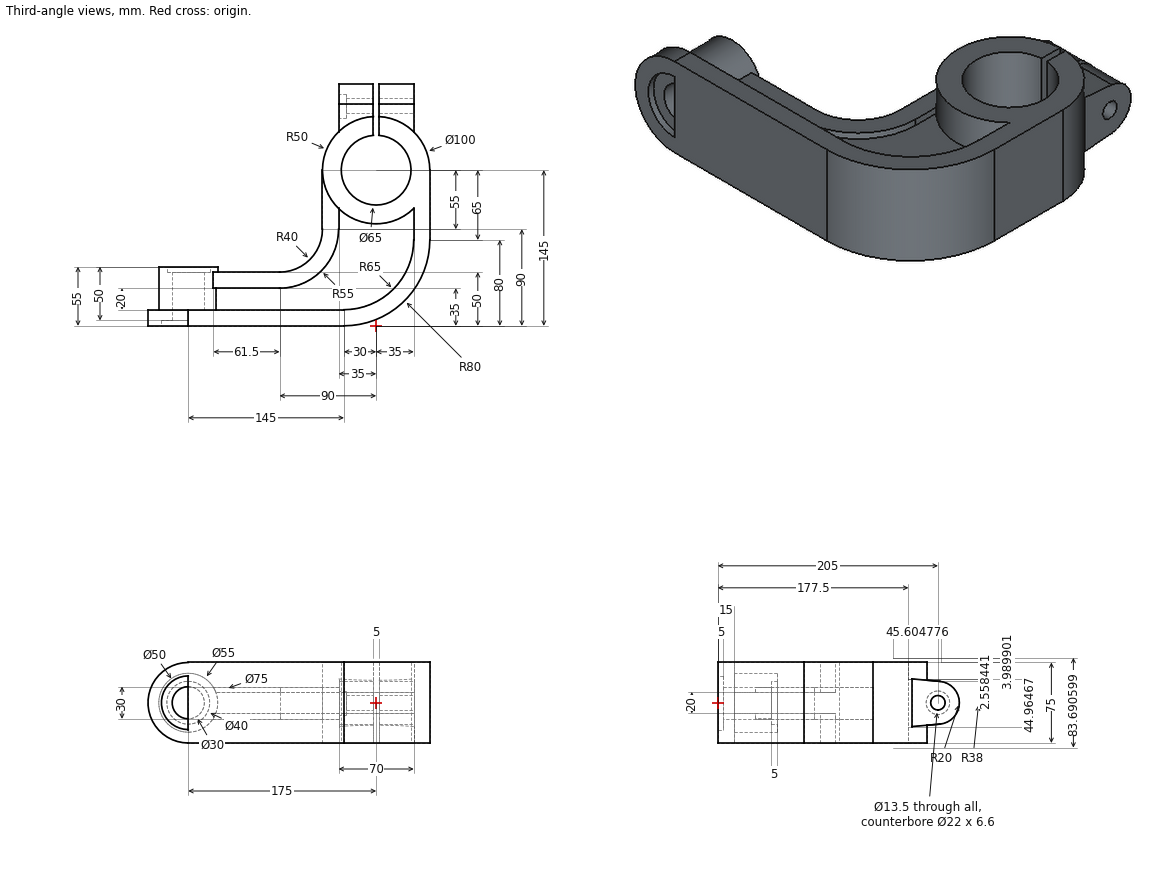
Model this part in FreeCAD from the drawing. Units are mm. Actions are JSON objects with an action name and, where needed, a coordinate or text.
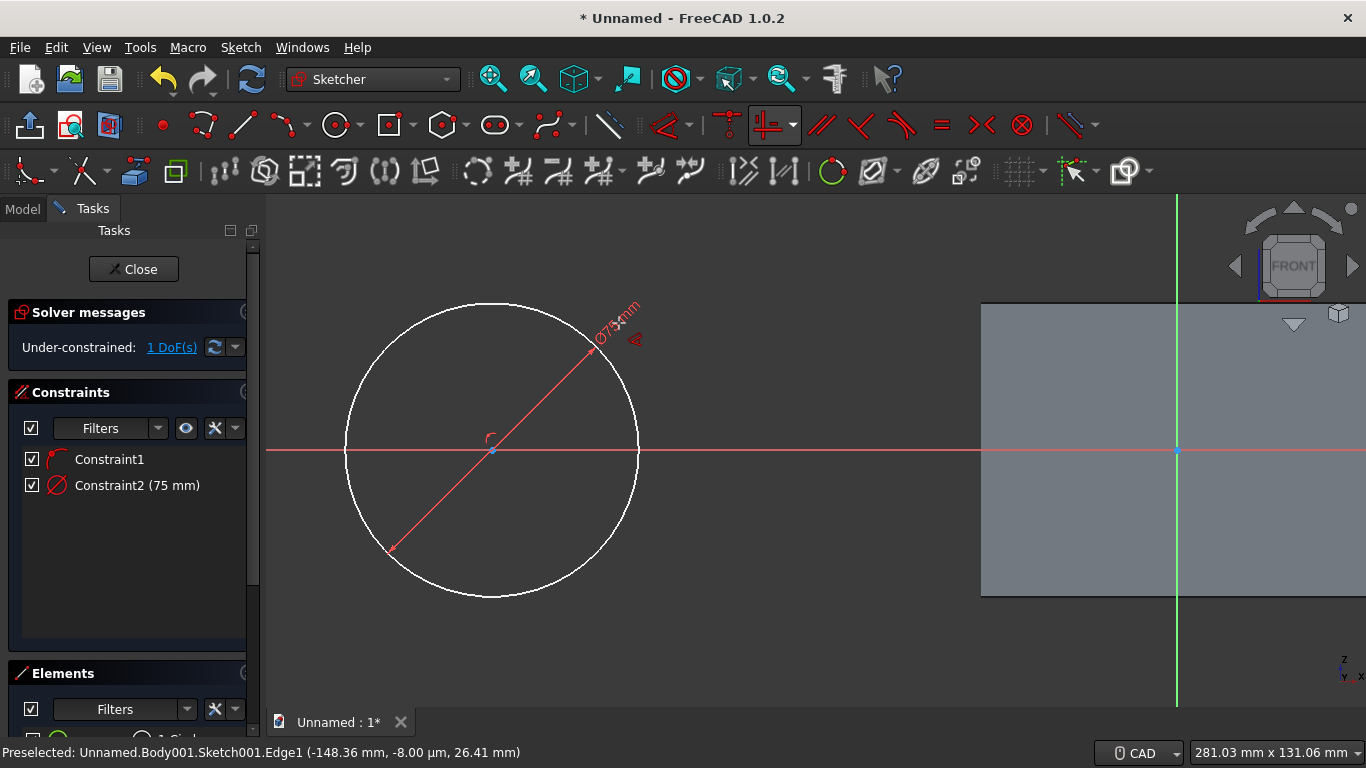
{"action": "left_click", "coordinate": [492, 450]}
{"action": "left_click", "coordinate": [835, 484]}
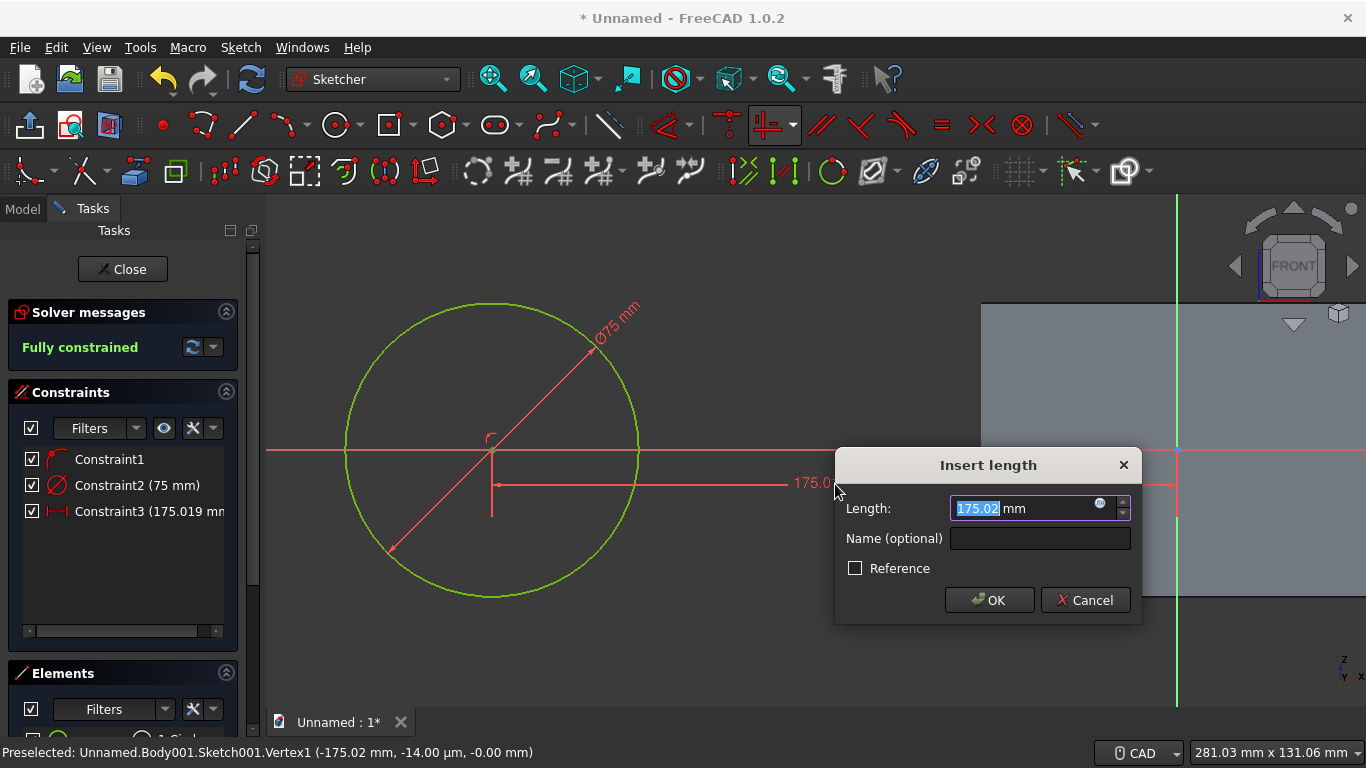
{"action": "type", "text": "175"}
{"action": "key", "text": "Return"}
{"action": "key", "text": "Escape"}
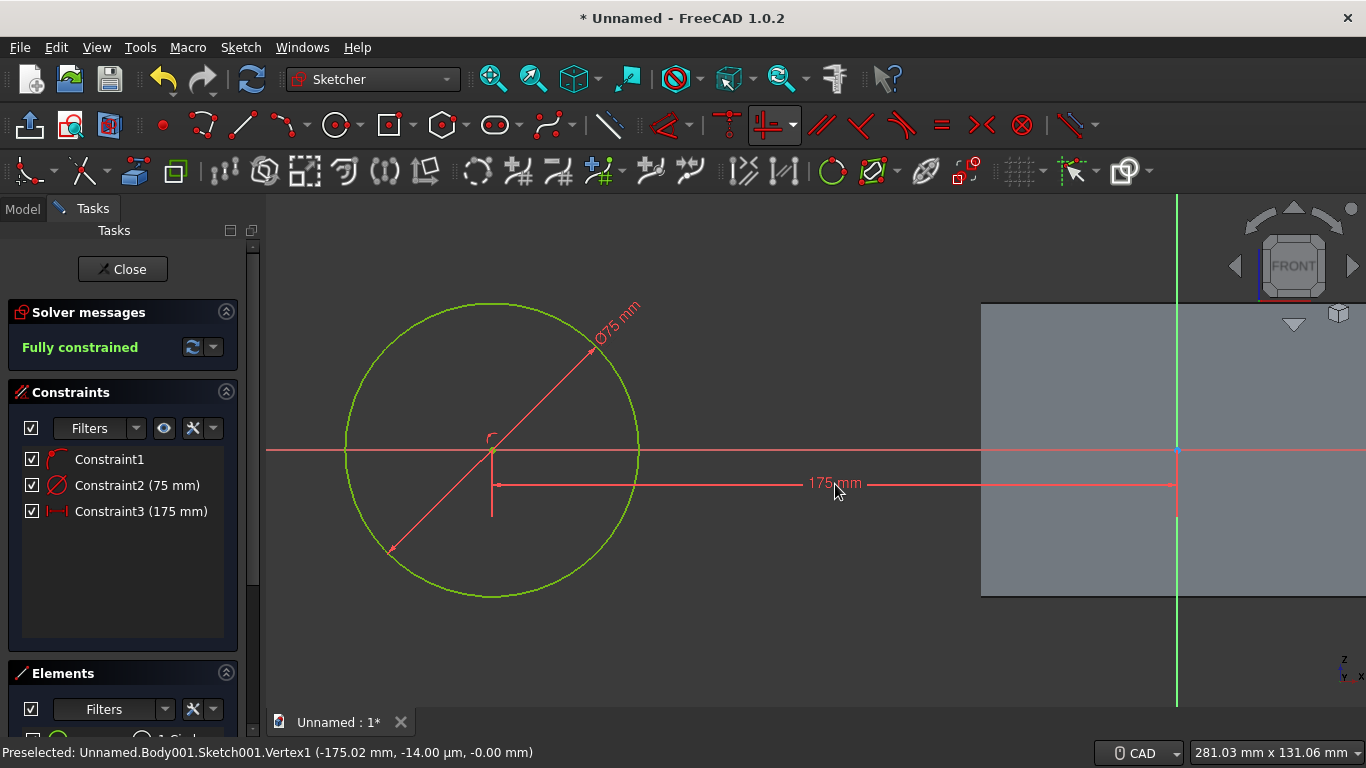
{"action": "left_click", "coordinate": [123, 269]}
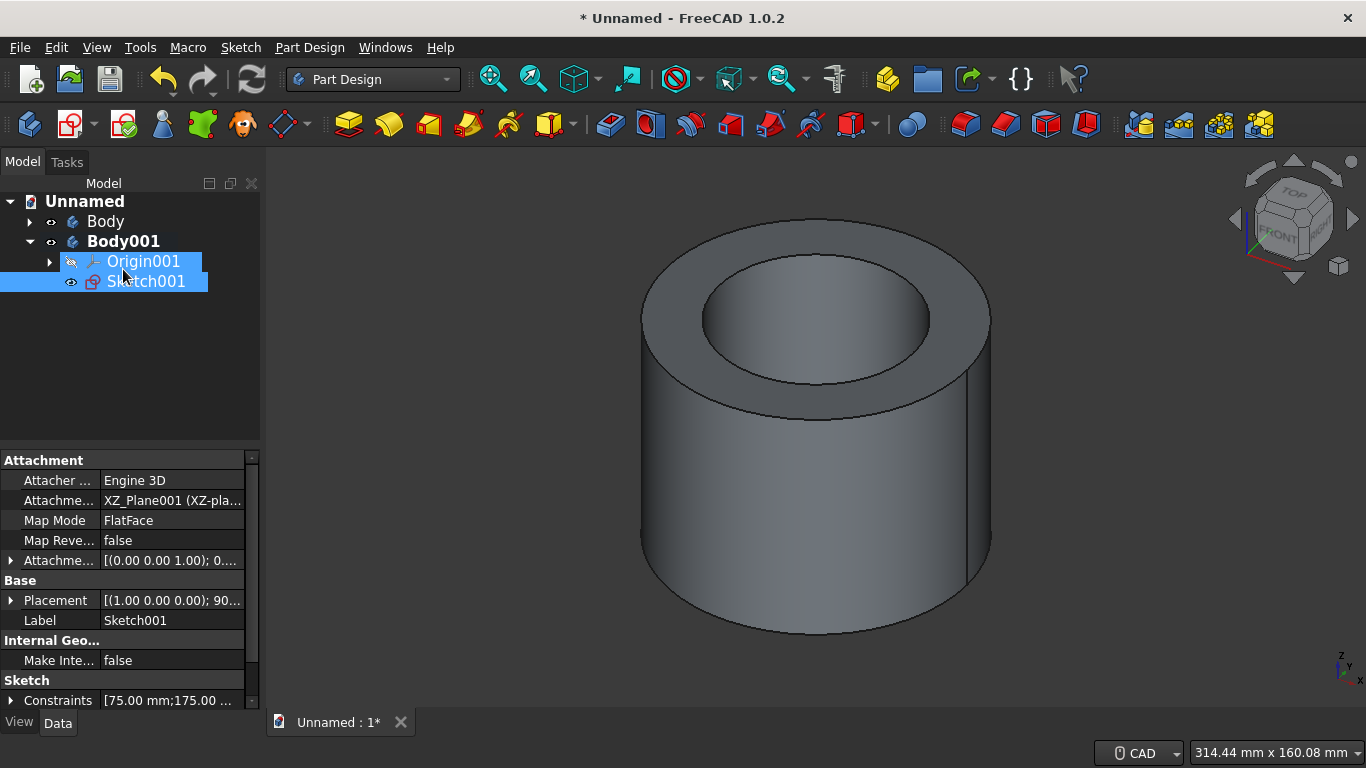
{"action": "left_click", "coordinate": [350, 124]}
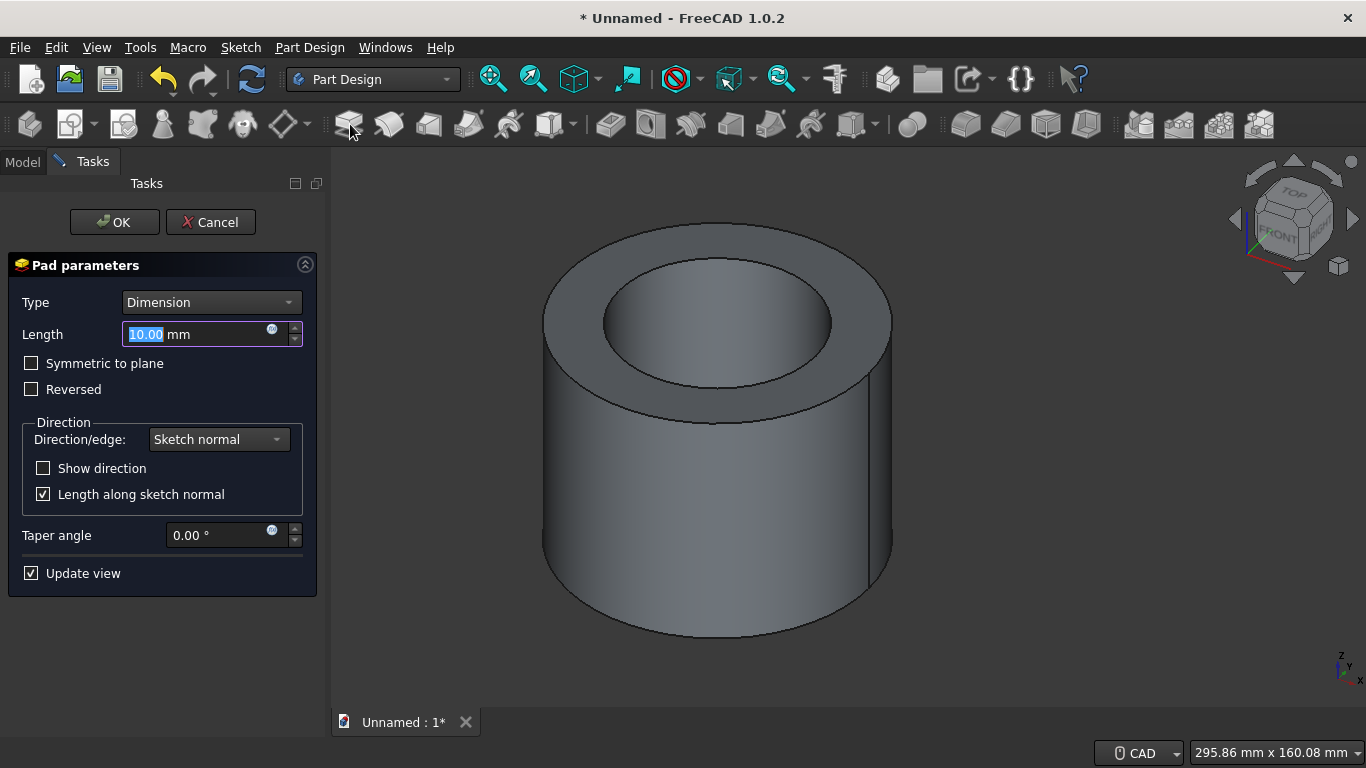
{"action": "type", "text": "15"}
{"action": "key", "text": "Tab"}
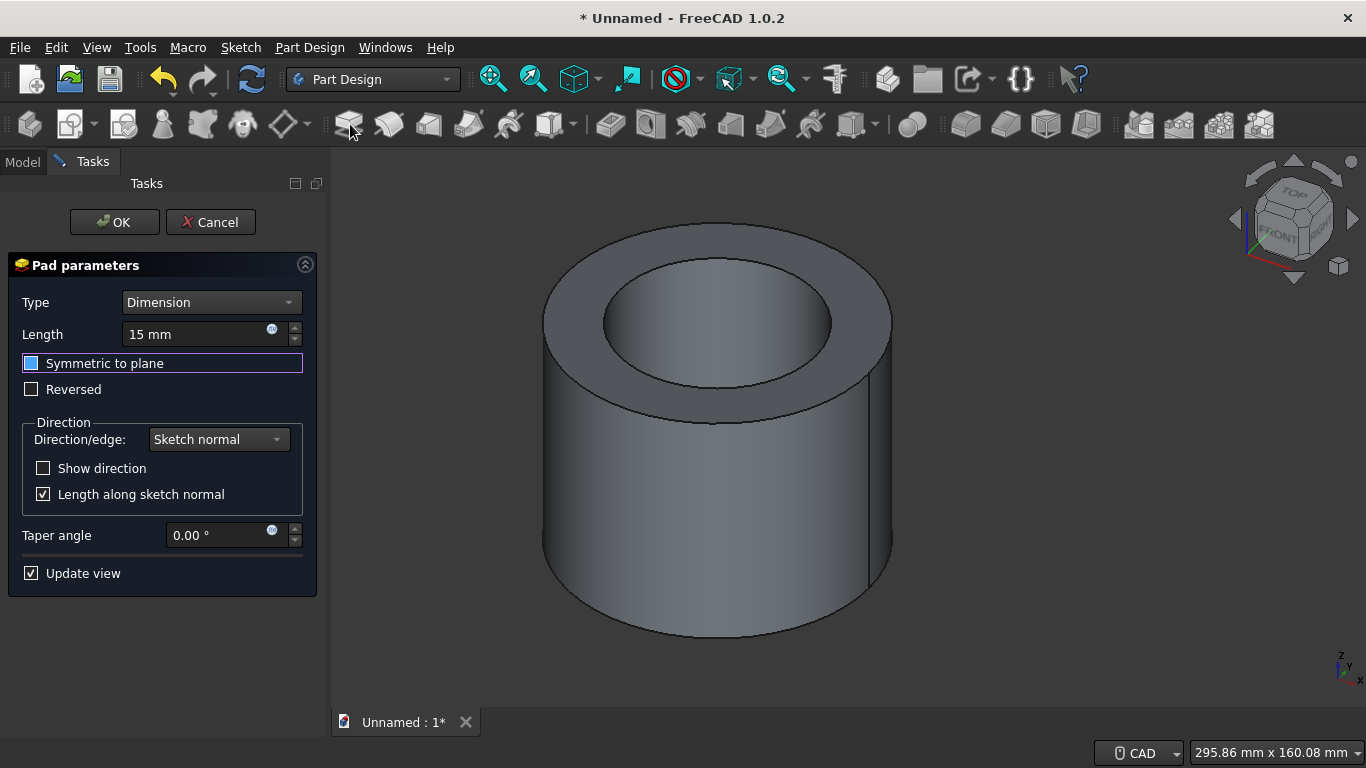
{"action": "left_click", "coordinate": [30, 389]}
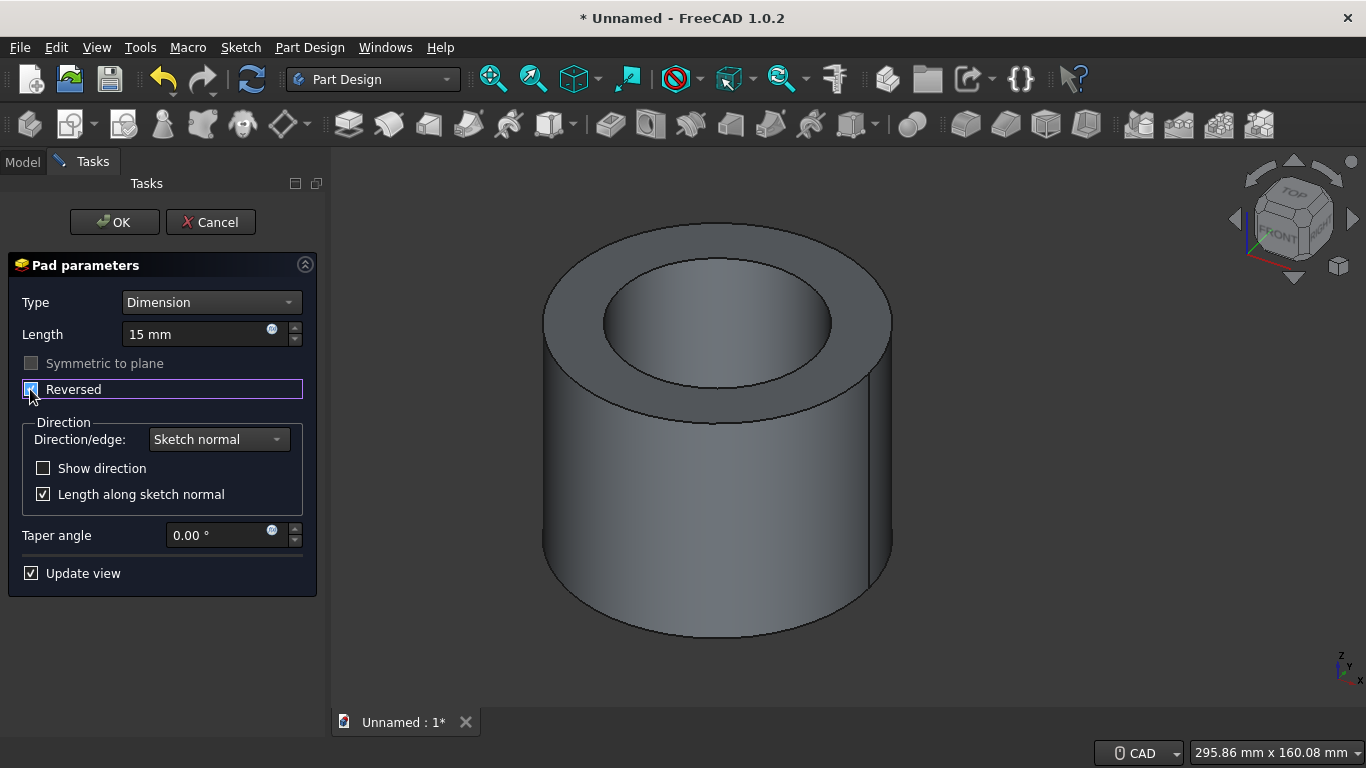
{"action": "left_click", "coordinate": [115, 222]}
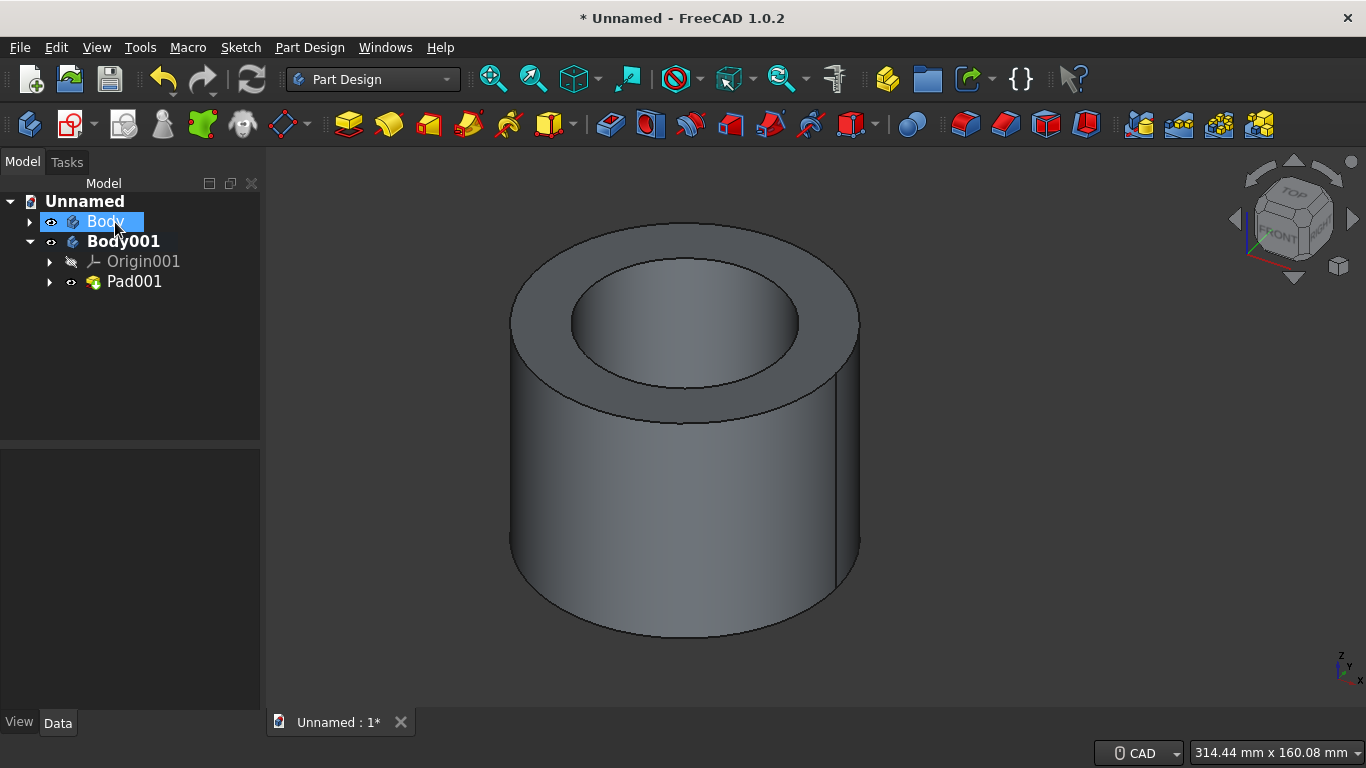
{"action": "key", "text": "v f"}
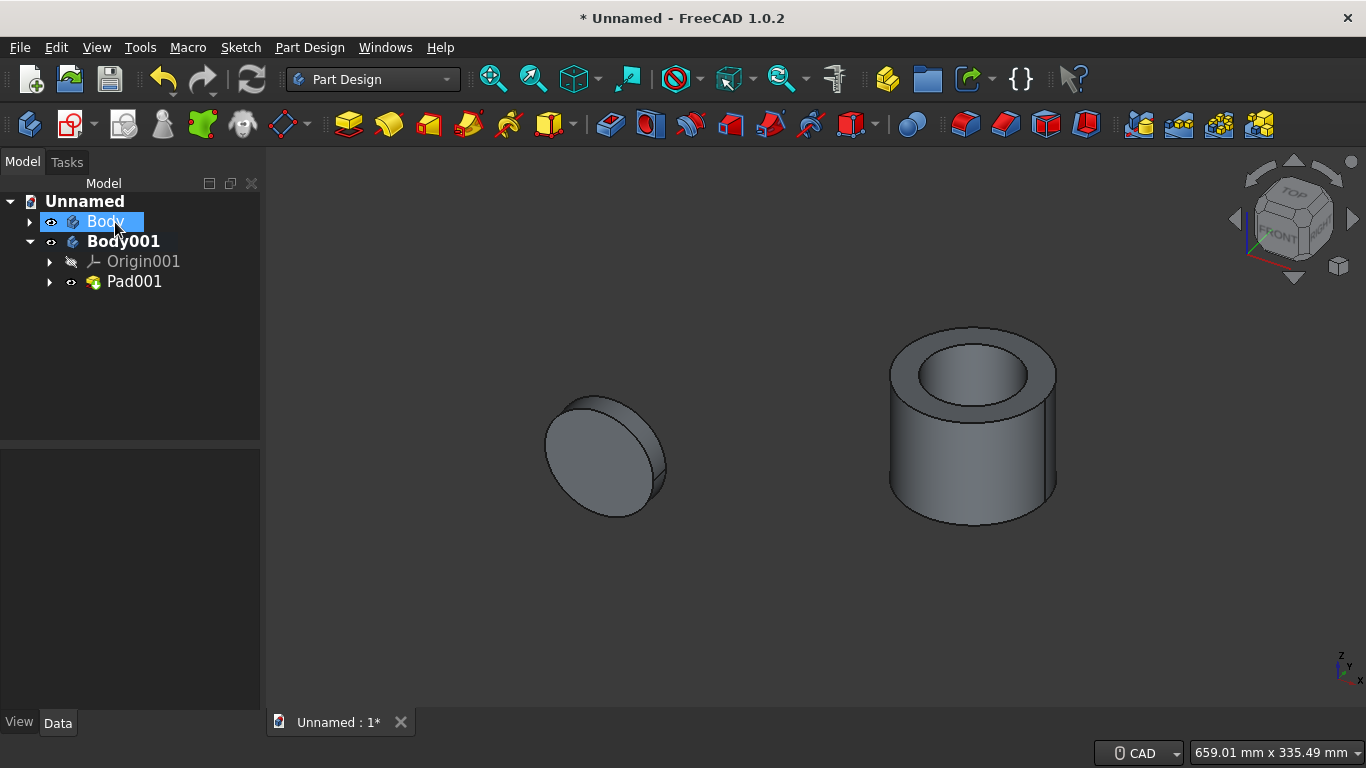
{"action": "left_click", "coordinate": [599, 462]}